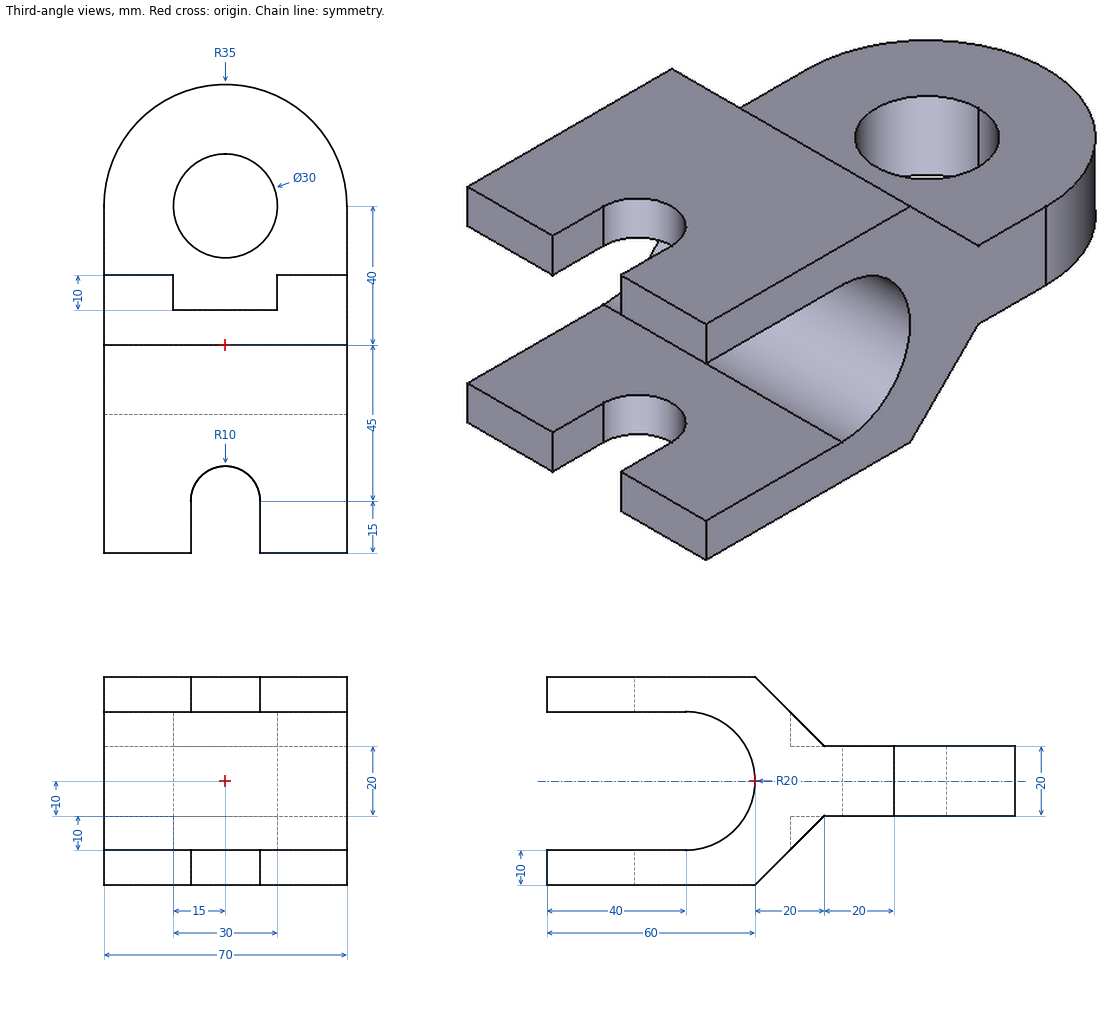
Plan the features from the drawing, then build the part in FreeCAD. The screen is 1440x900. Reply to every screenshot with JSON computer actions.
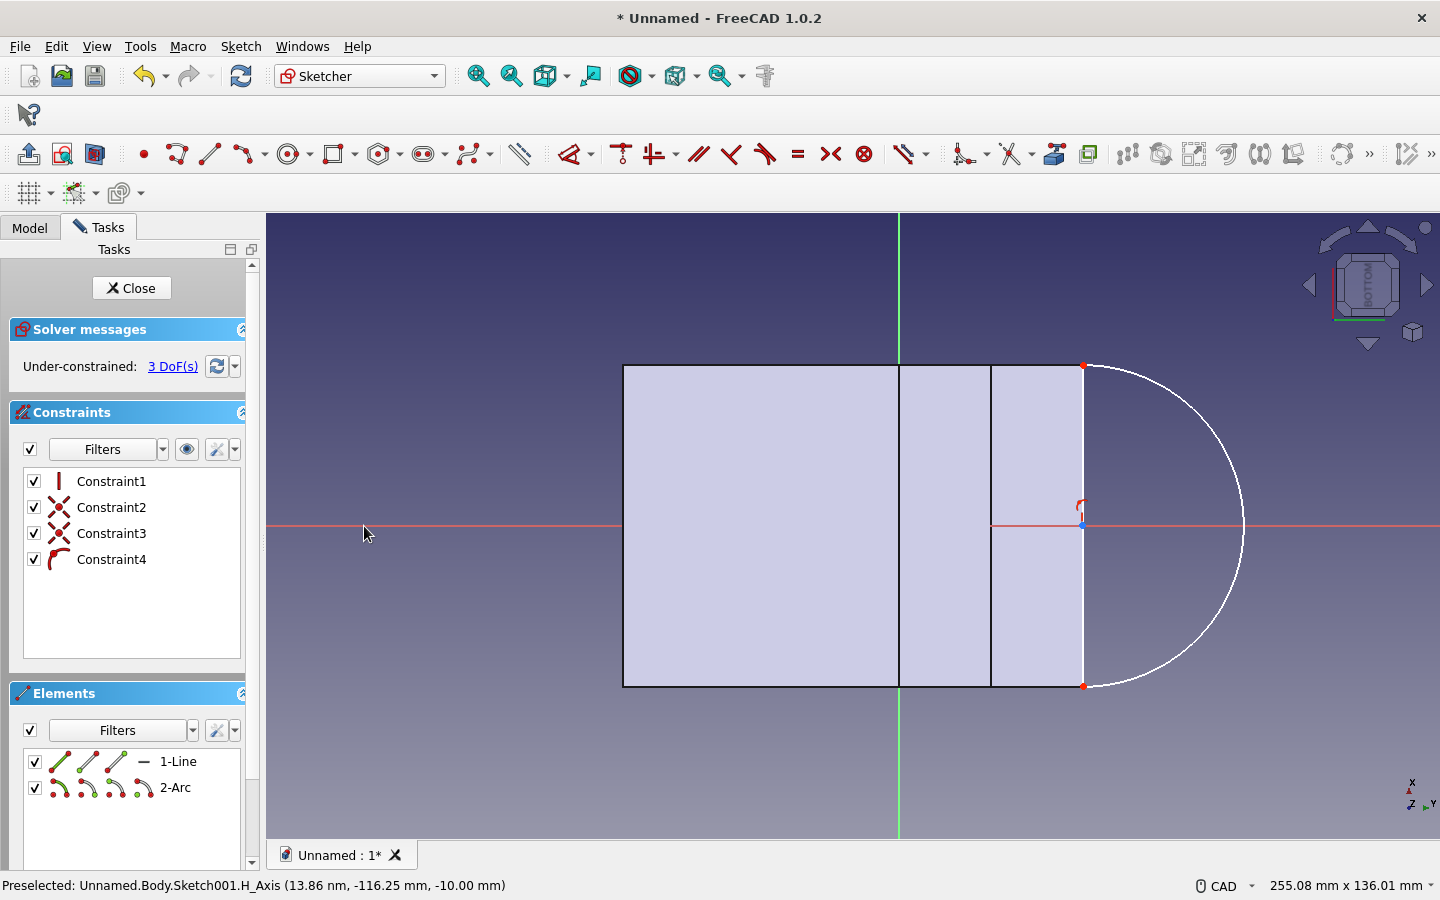
{"action": "left_click", "coordinate": [568, 154]}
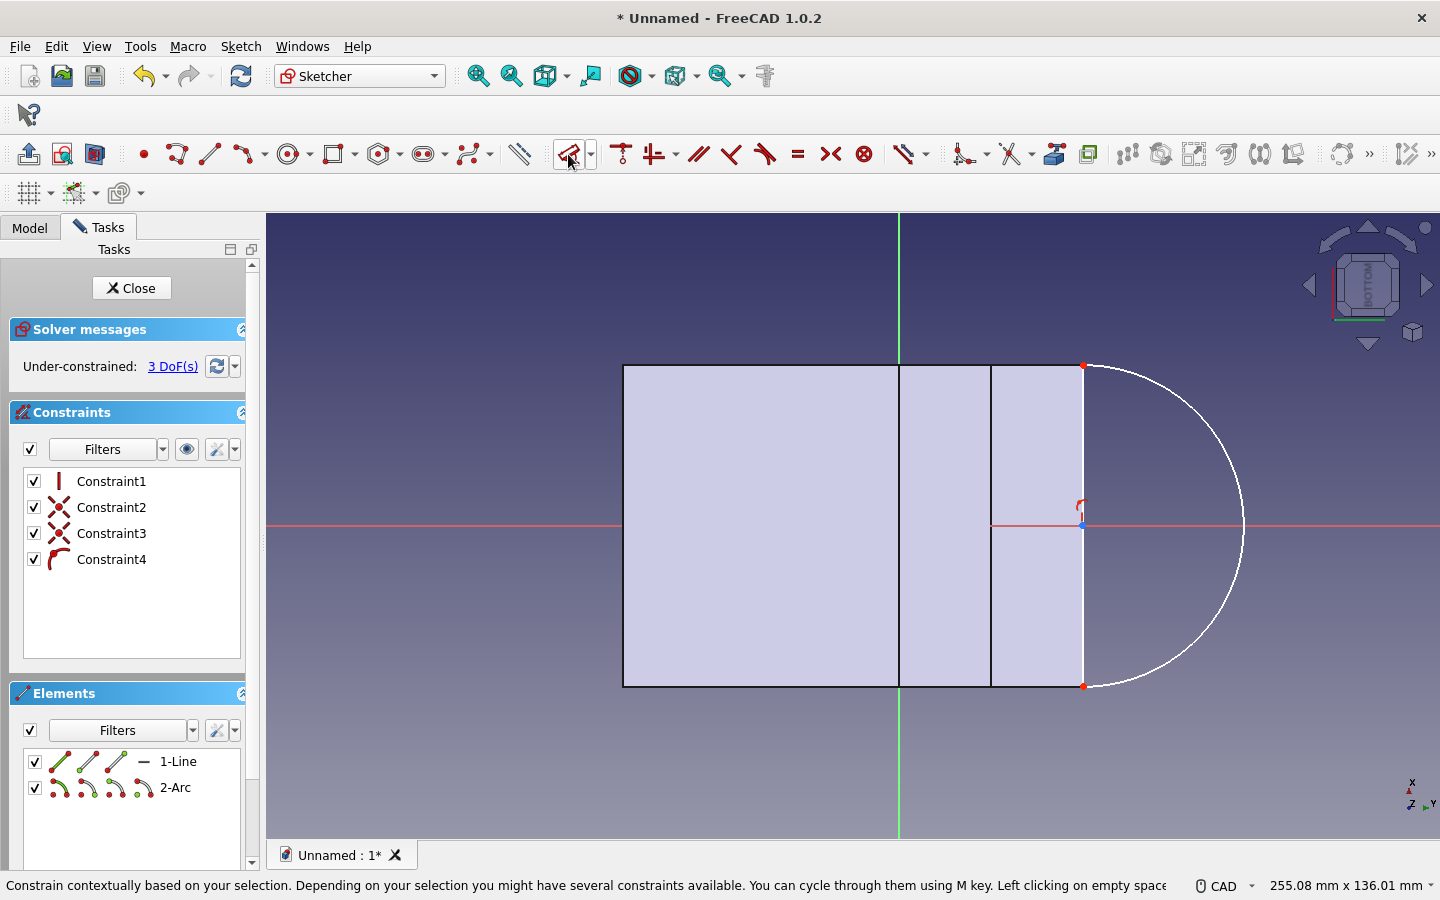
{"action": "left_click", "coordinate": [1213, 621]}
{"action": "left_click", "coordinate": [1239, 640]}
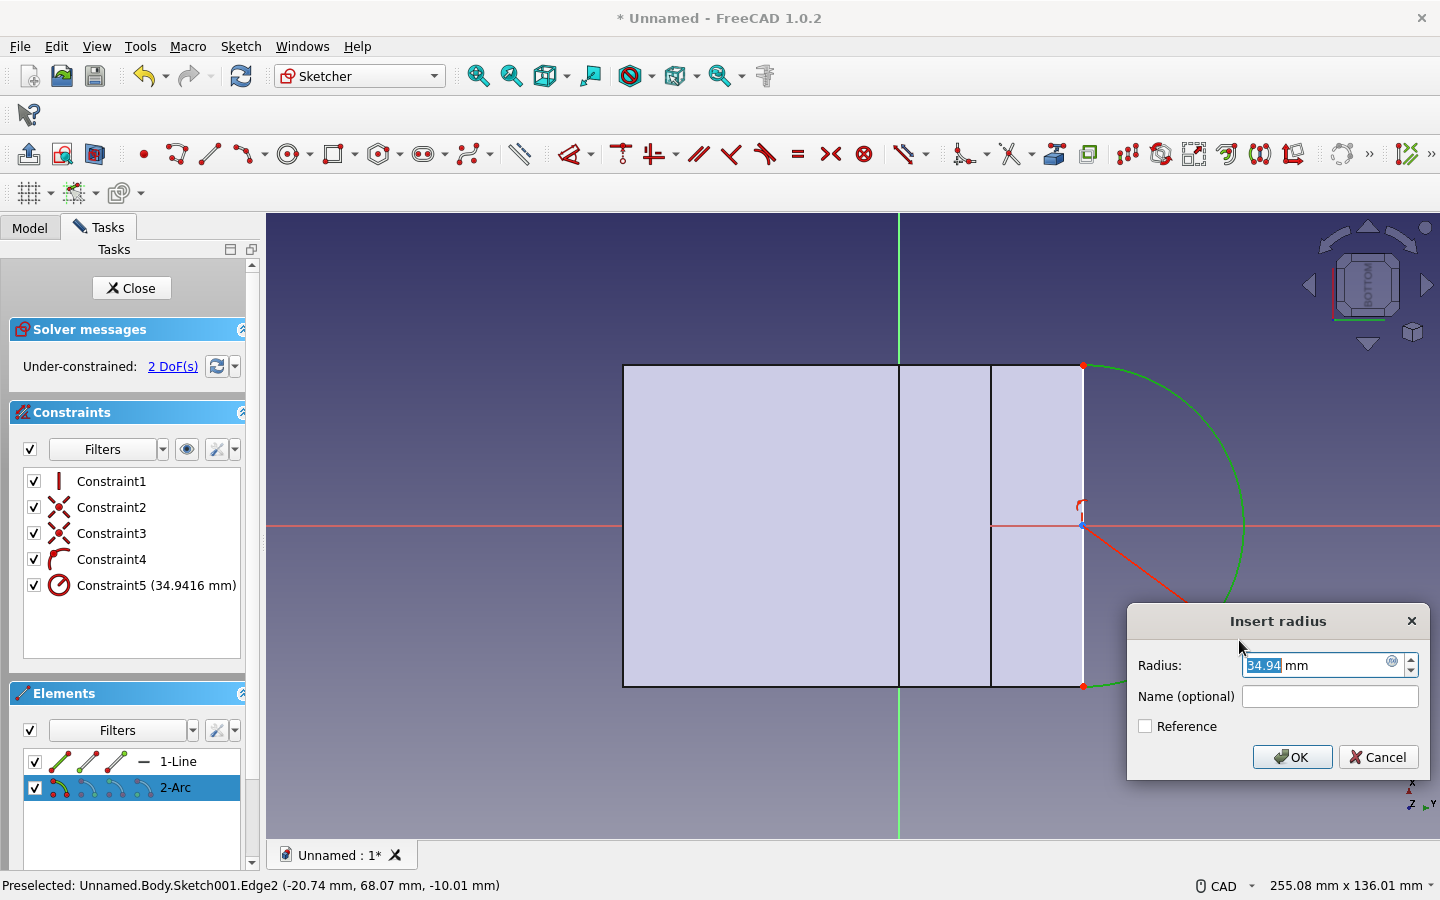
{"action": "type", "text": "35"}
{"action": "key", "text": "Return"}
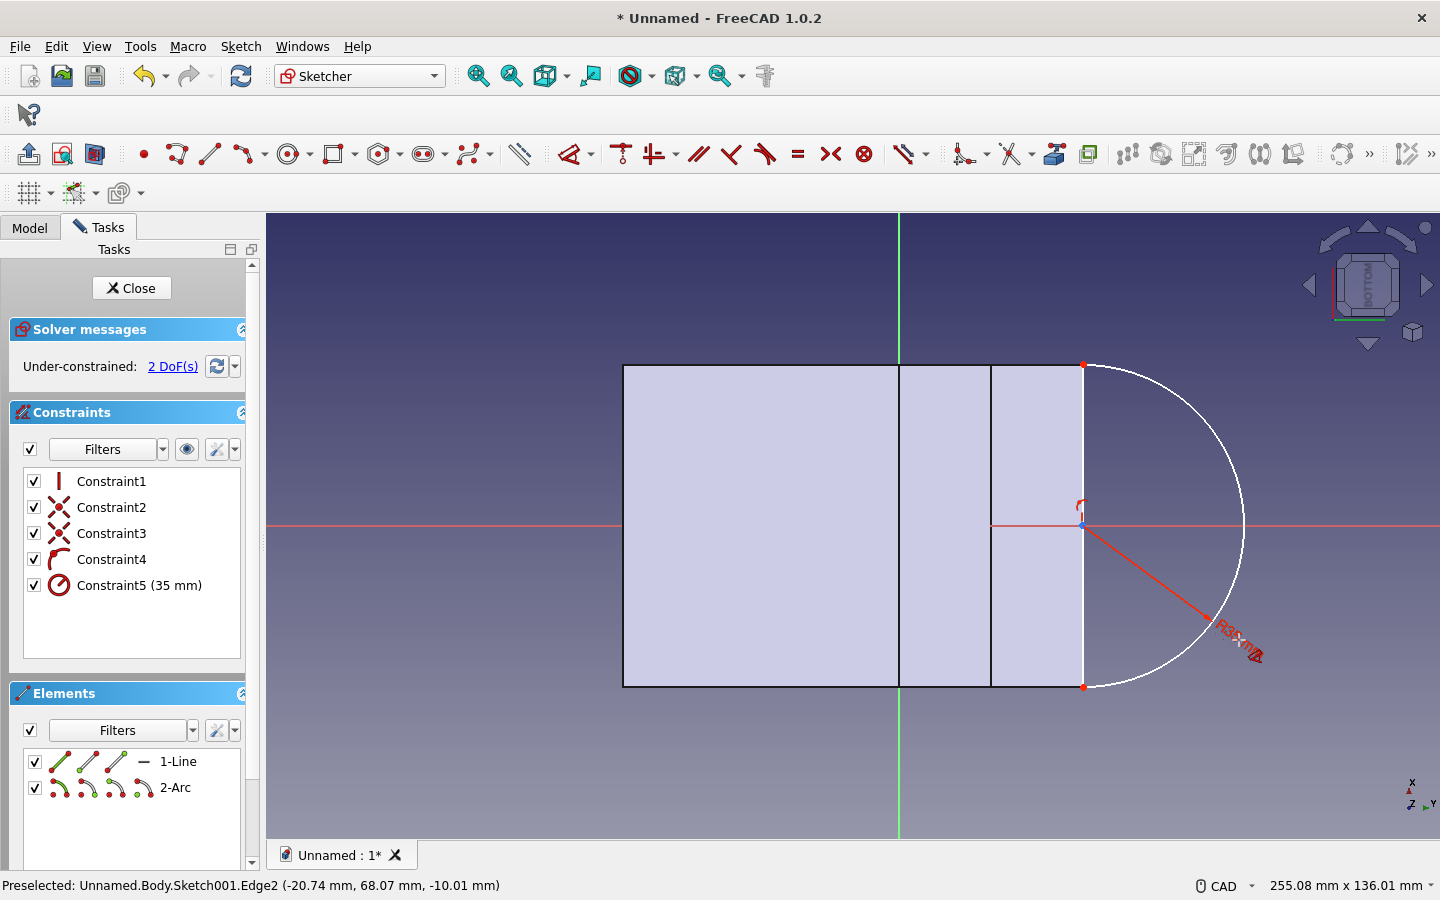
{"action": "left_click", "coordinate": [1083, 365]}
{"action": "left_click", "coordinate": [991, 331]}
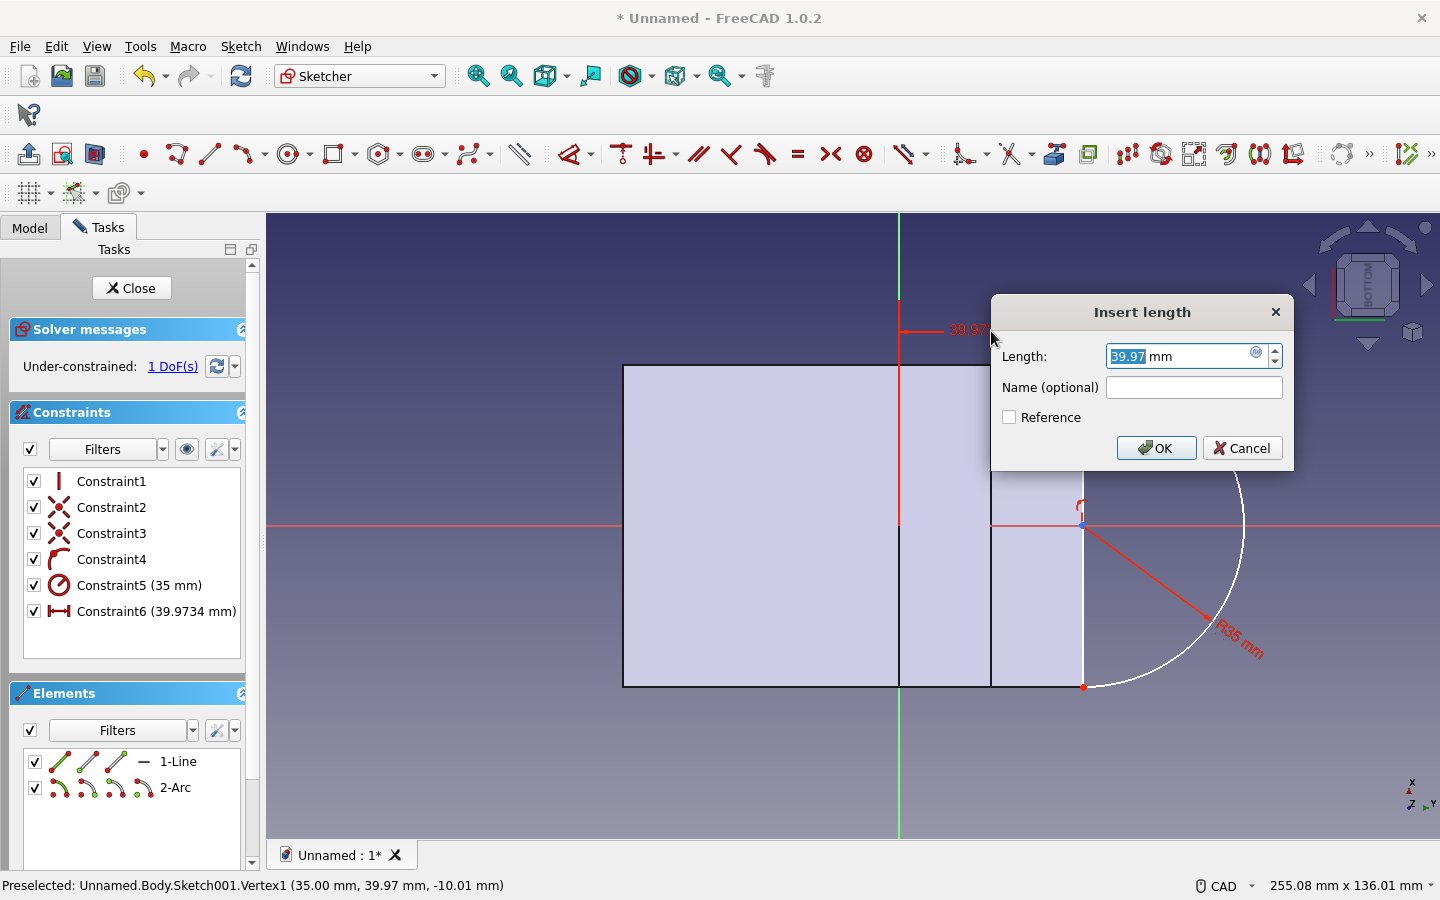
{"action": "type", "text": "40"}
{"action": "key", "text": "Return"}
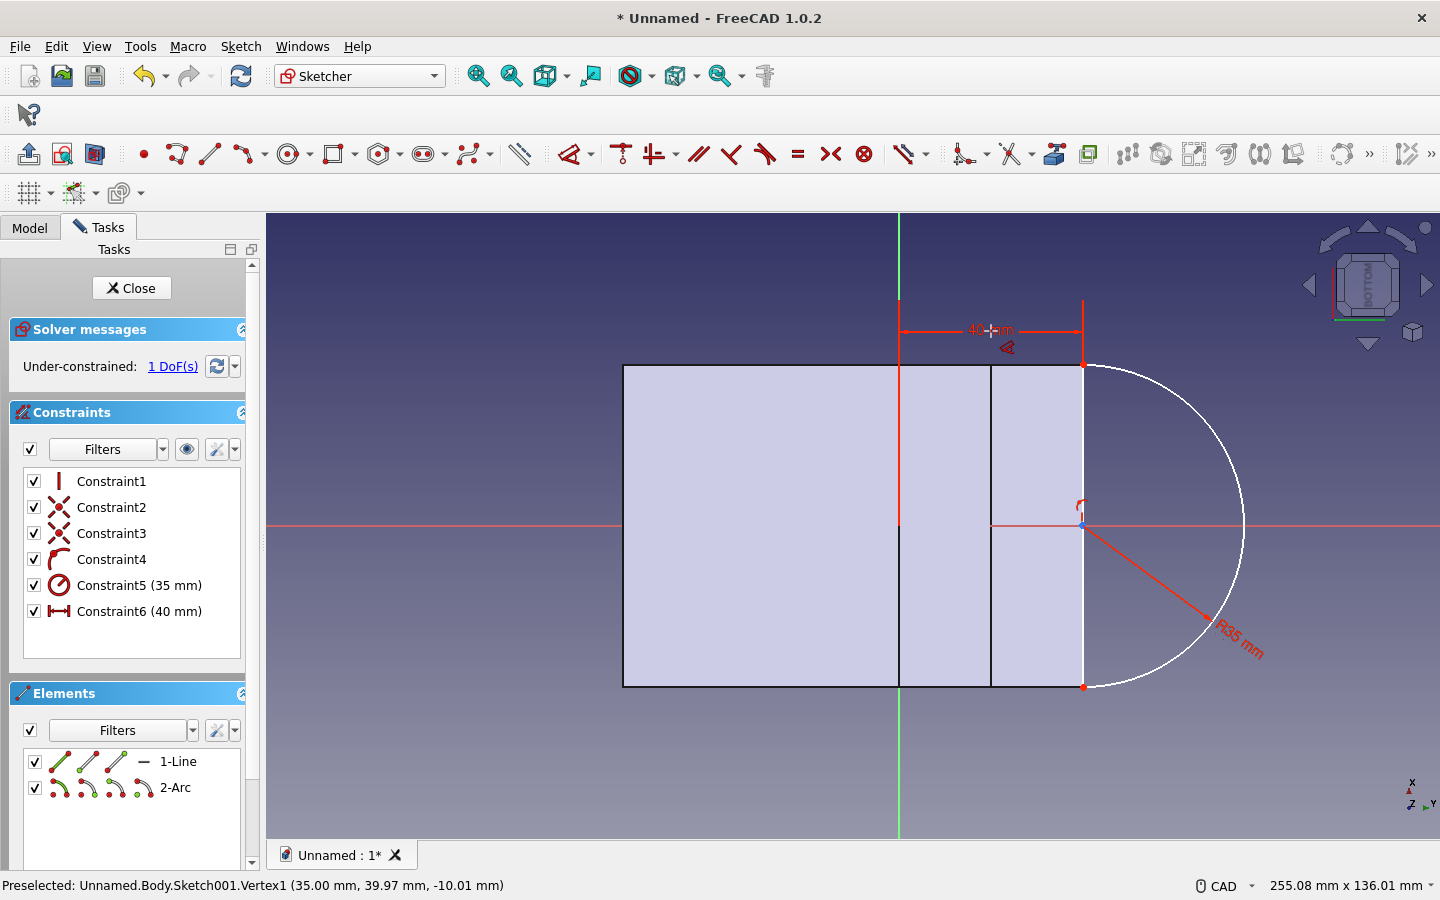
{"action": "left_click", "coordinate": [1083, 526]}
{"action": "left_click", "coordinate": [991, 560]}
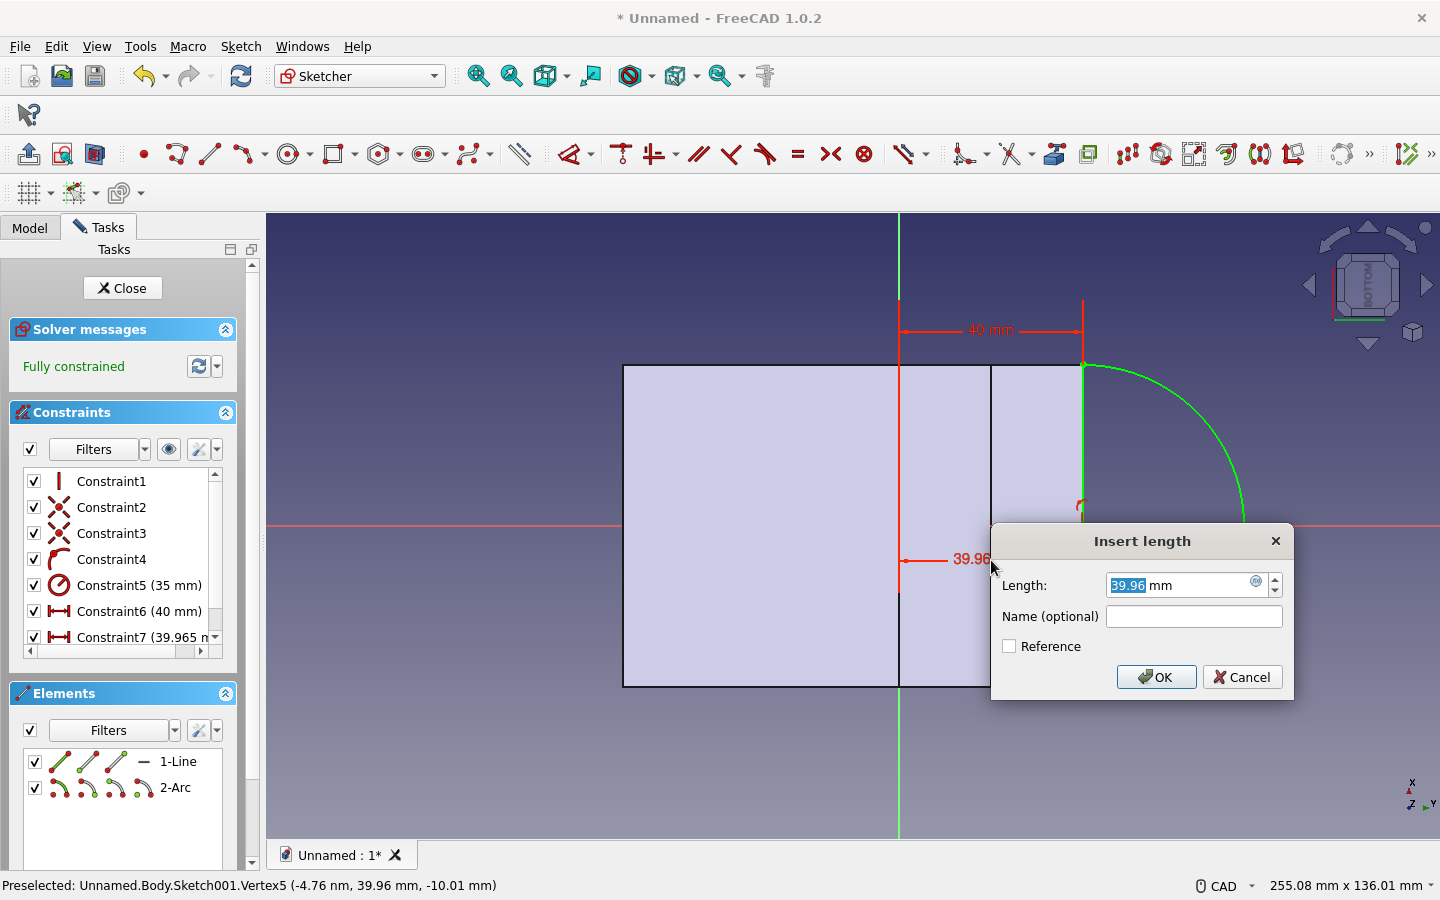
{"action": "type", "text": "40"}
{"action": "key", "text": "Return"}
{"action": "key", "text": "Escape"}